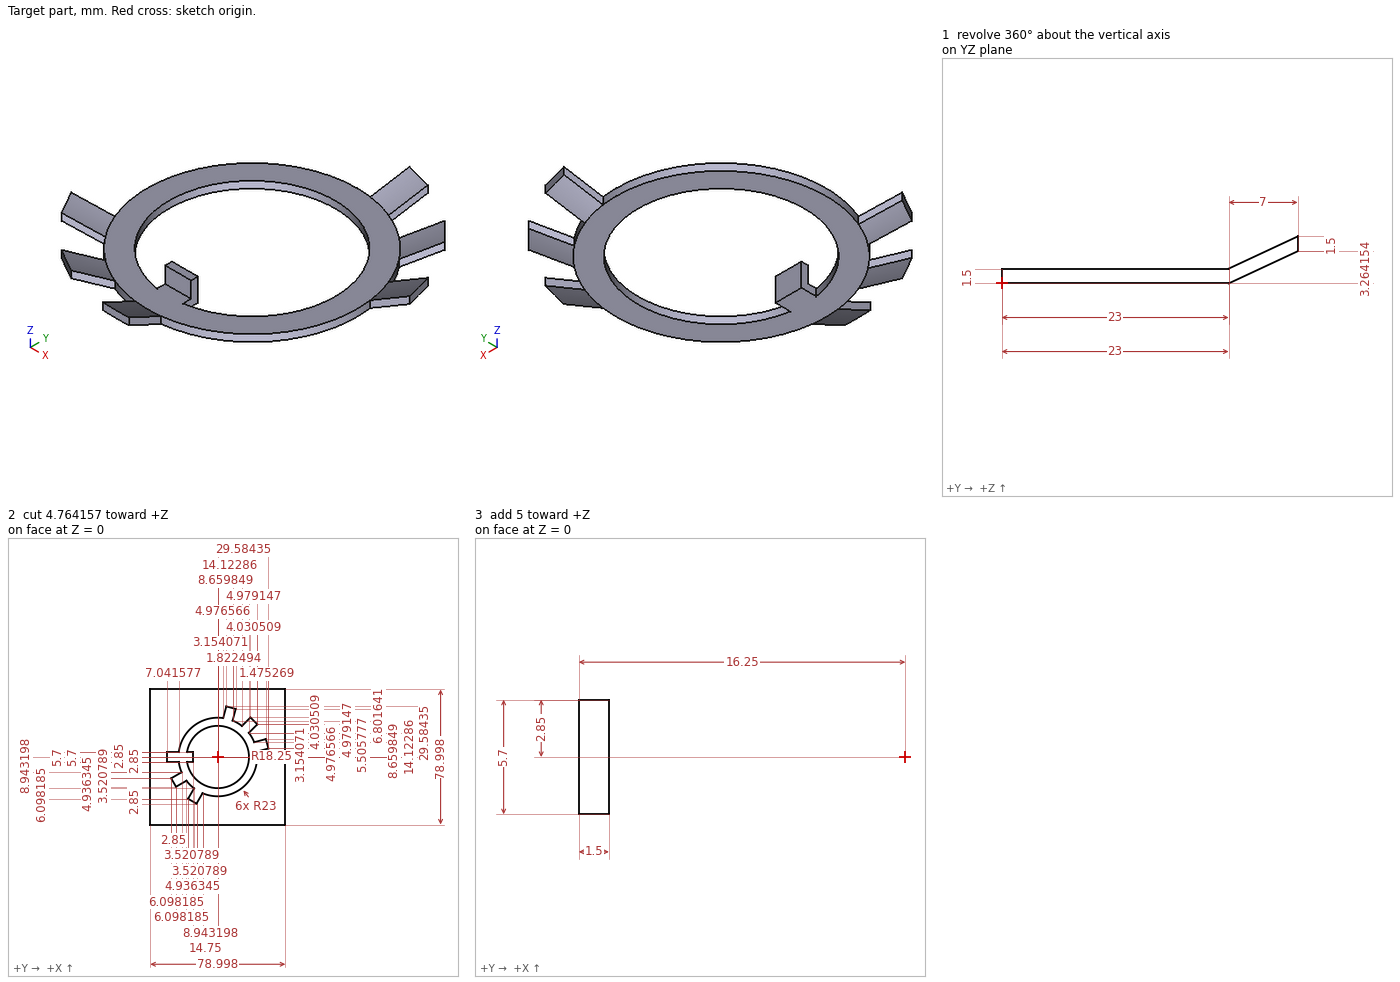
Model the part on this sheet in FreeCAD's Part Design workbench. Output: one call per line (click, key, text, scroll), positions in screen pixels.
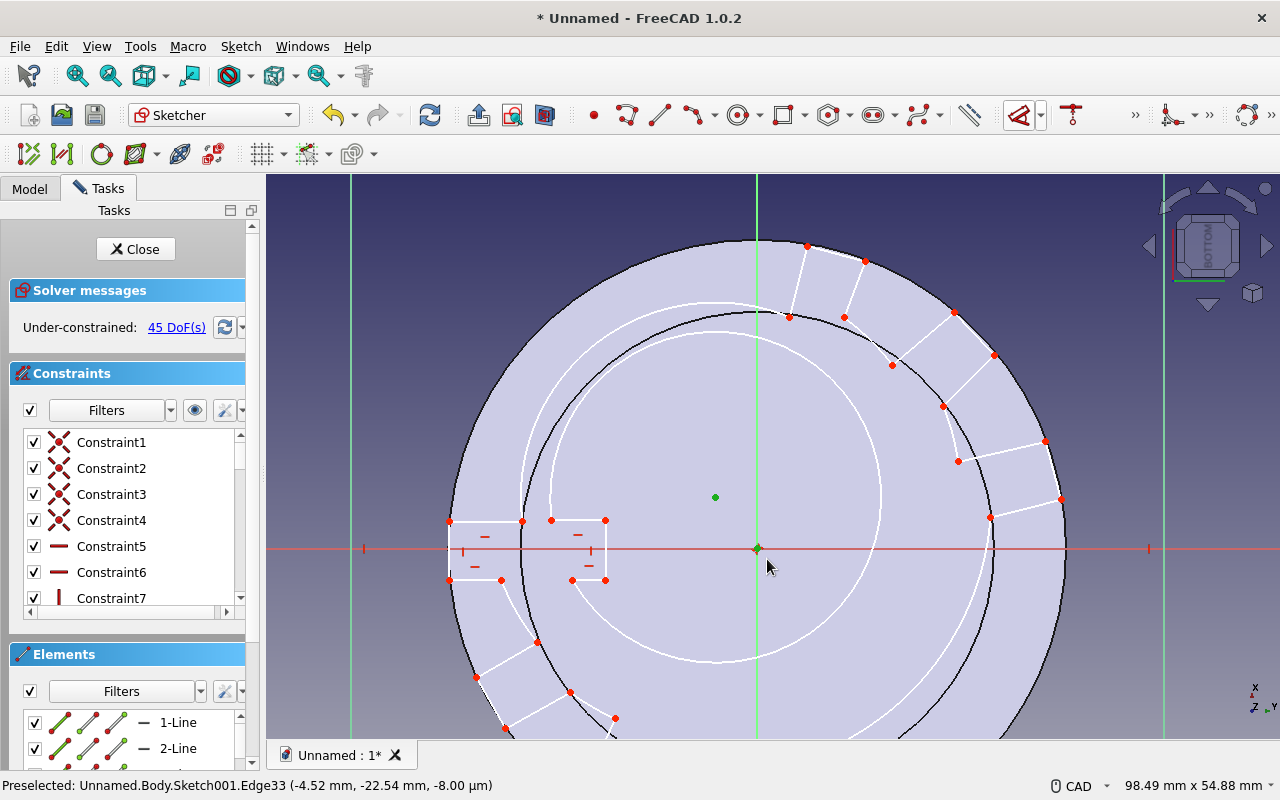
click(1071, 116)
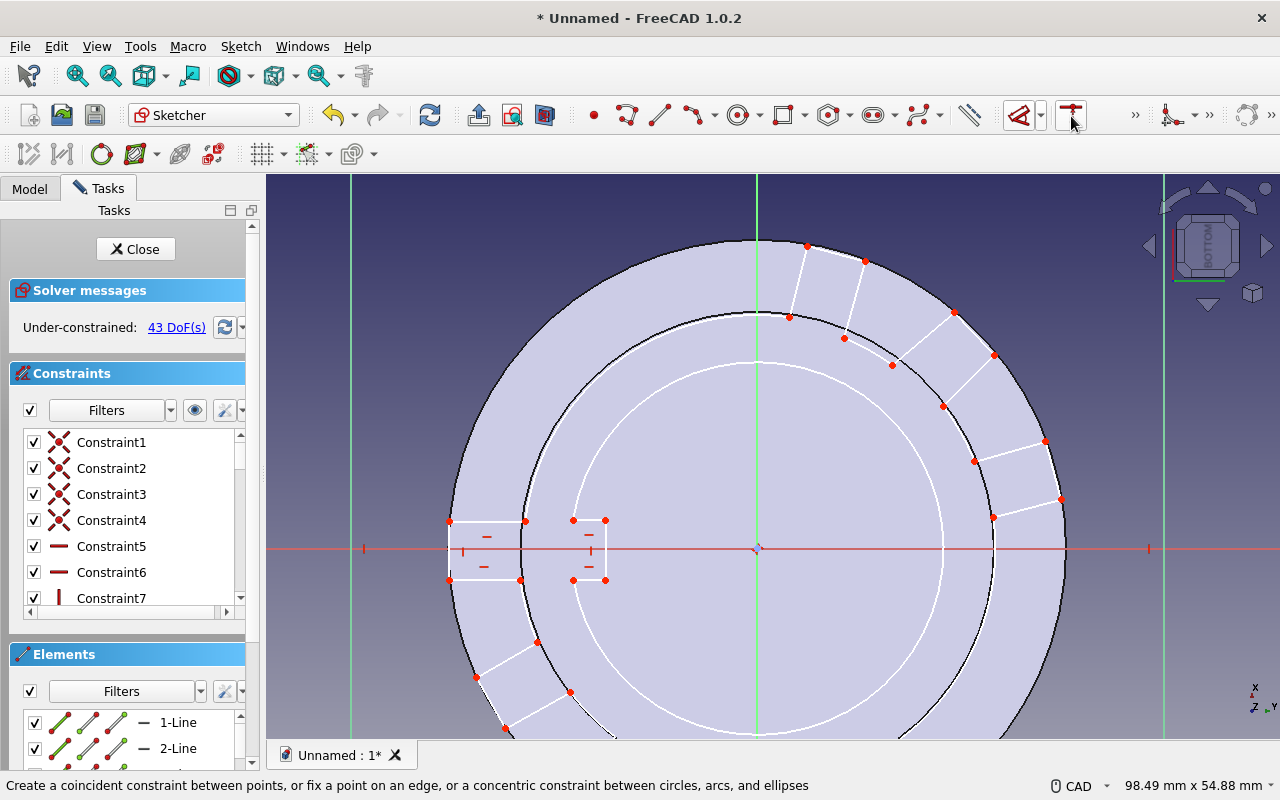
click(583, 707)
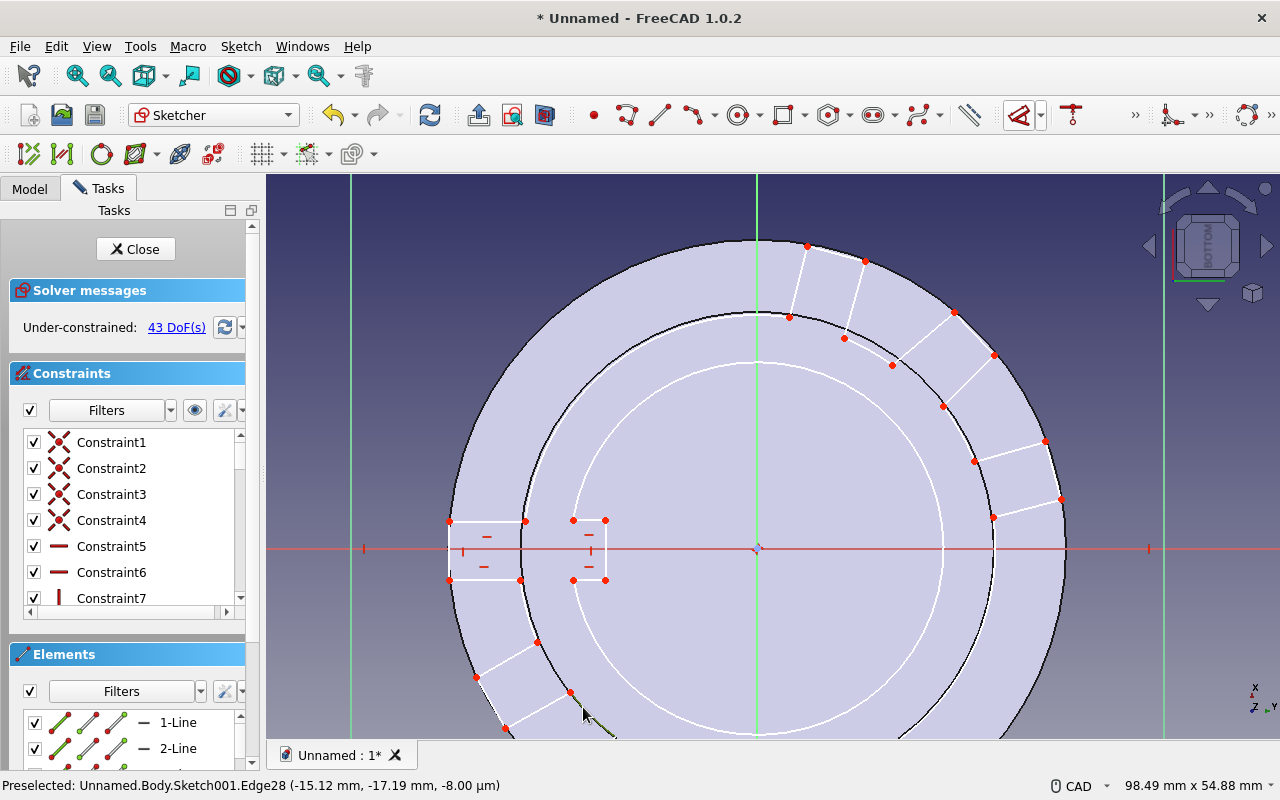
click(966, 662)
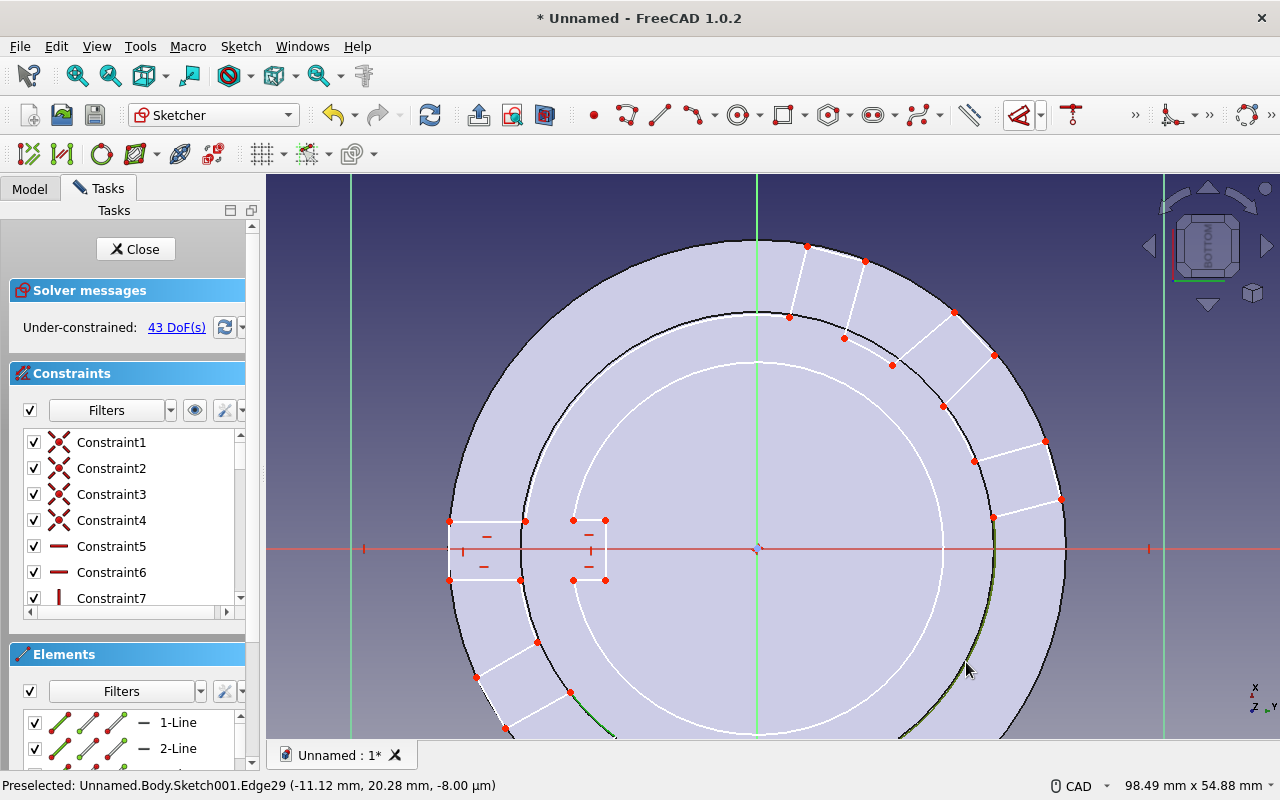
click(967, 444)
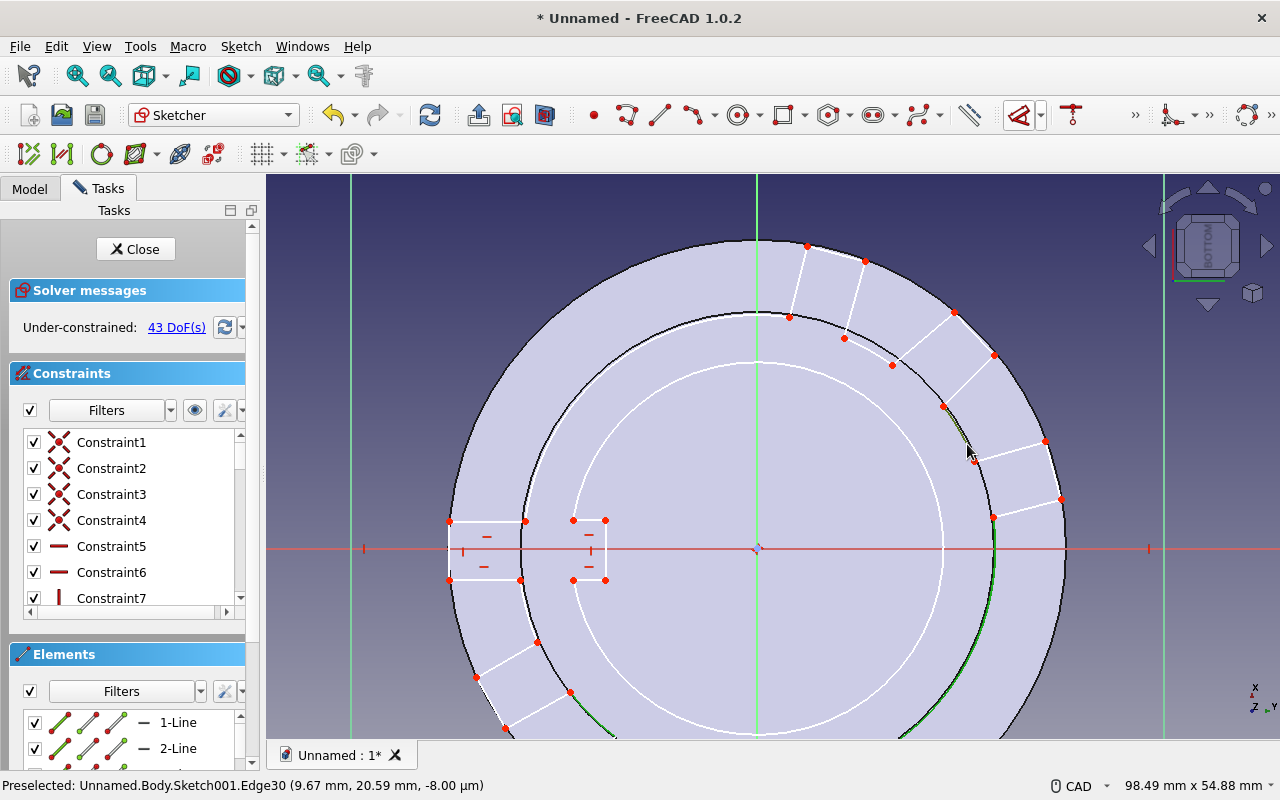
click(879, 356)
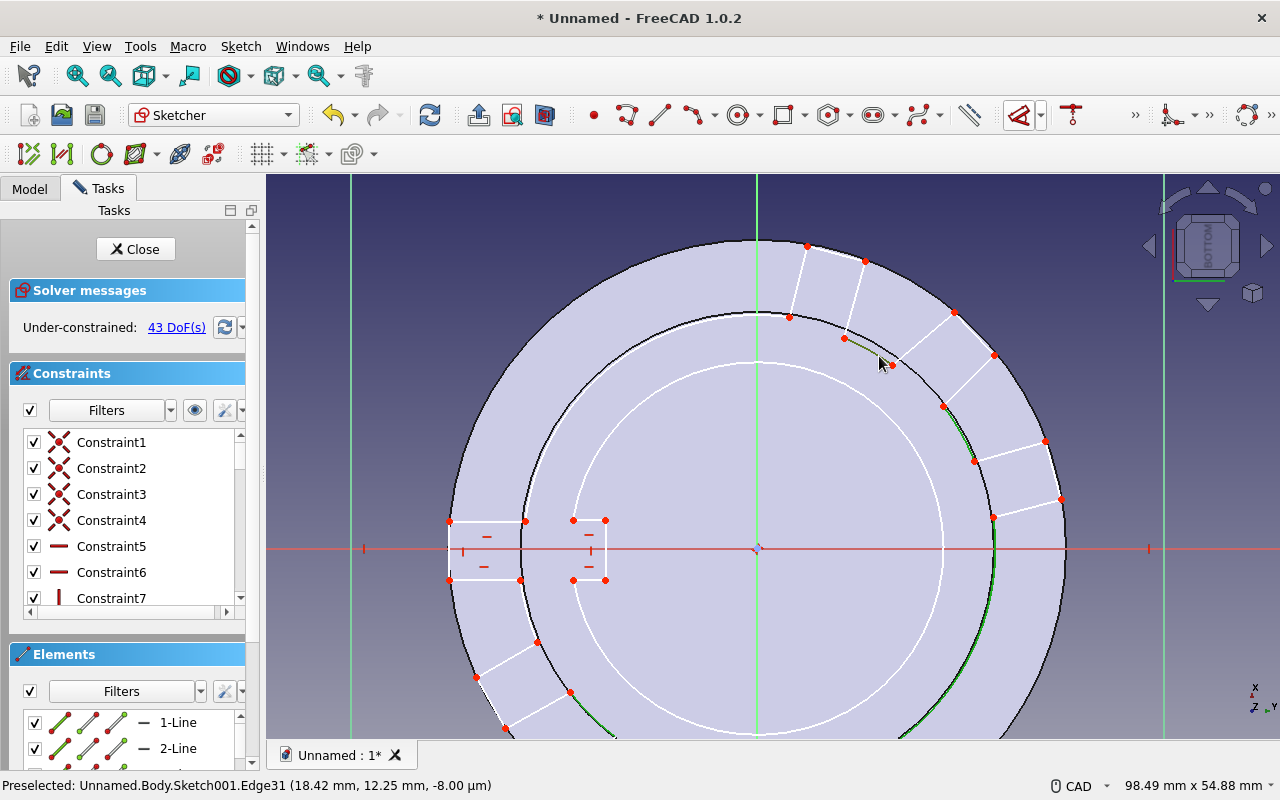
click(679, 328)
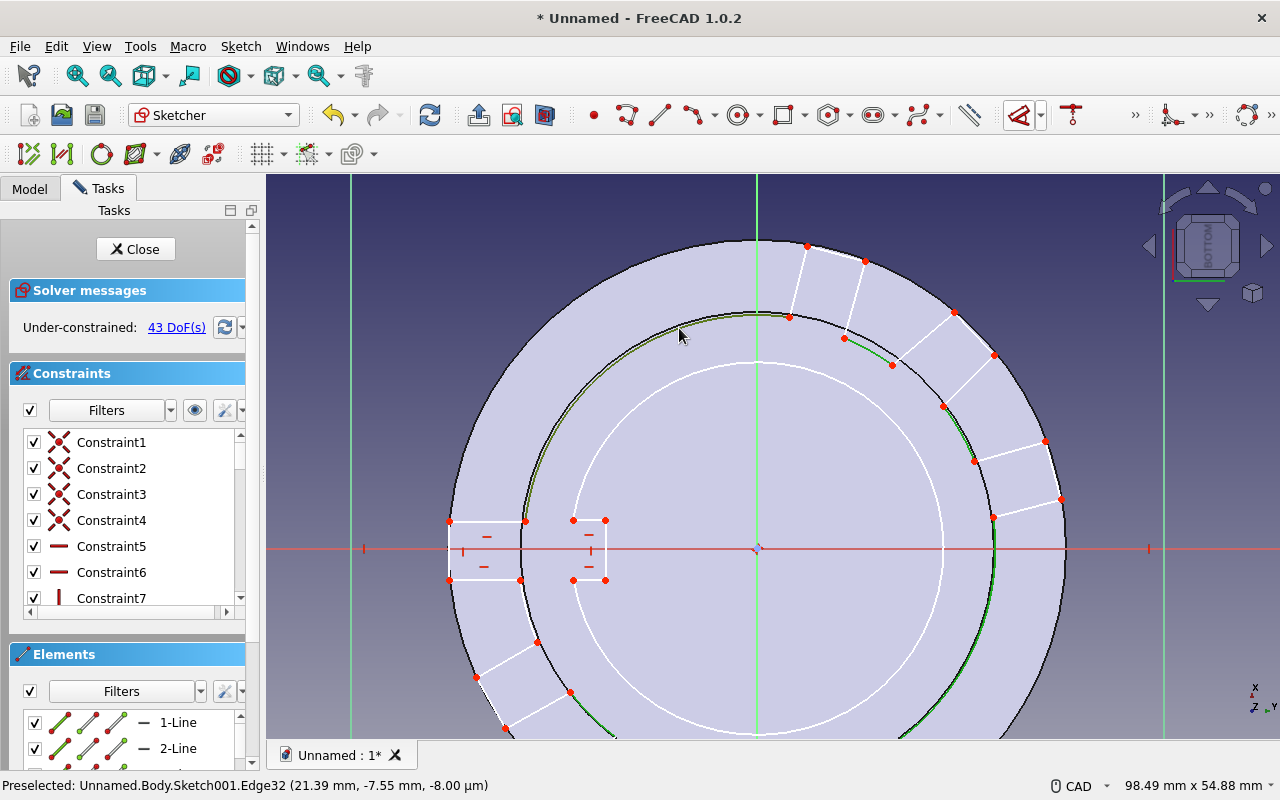
click(524, 600)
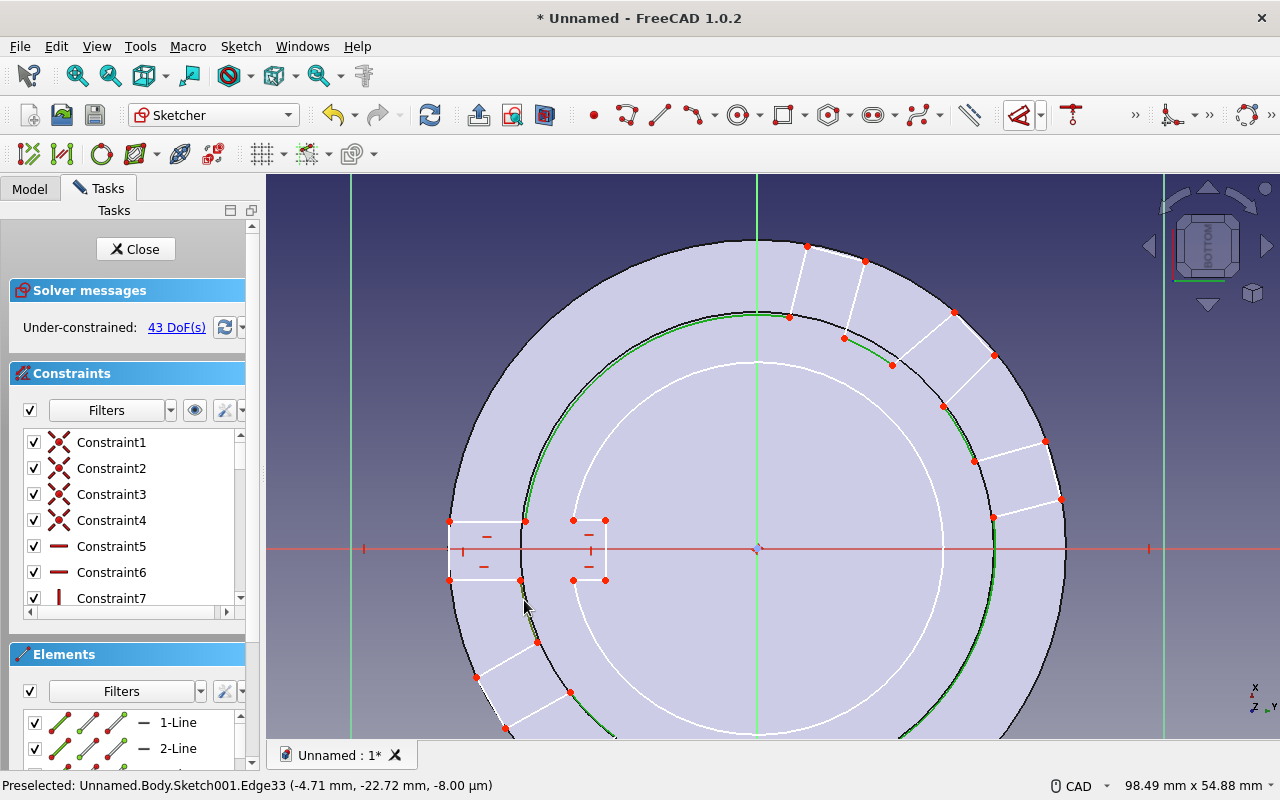
key(e)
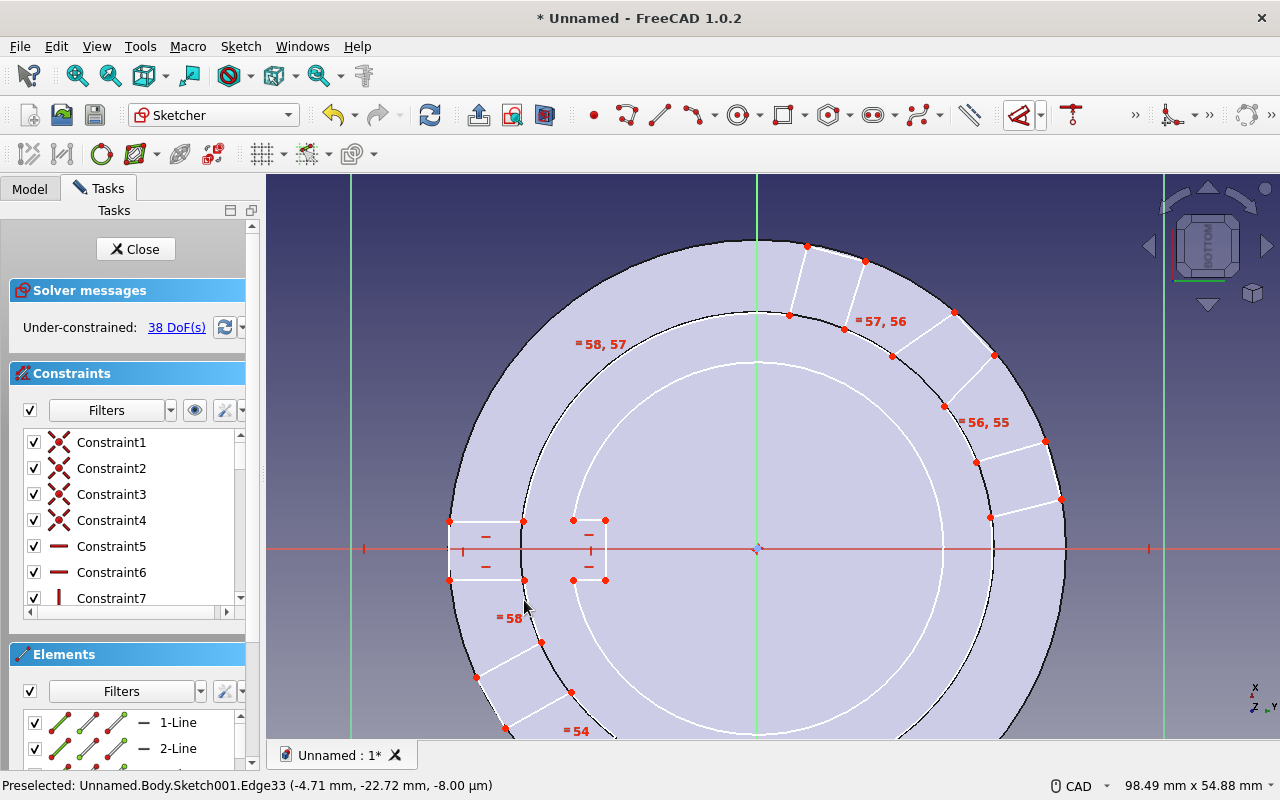
click(825, 375)